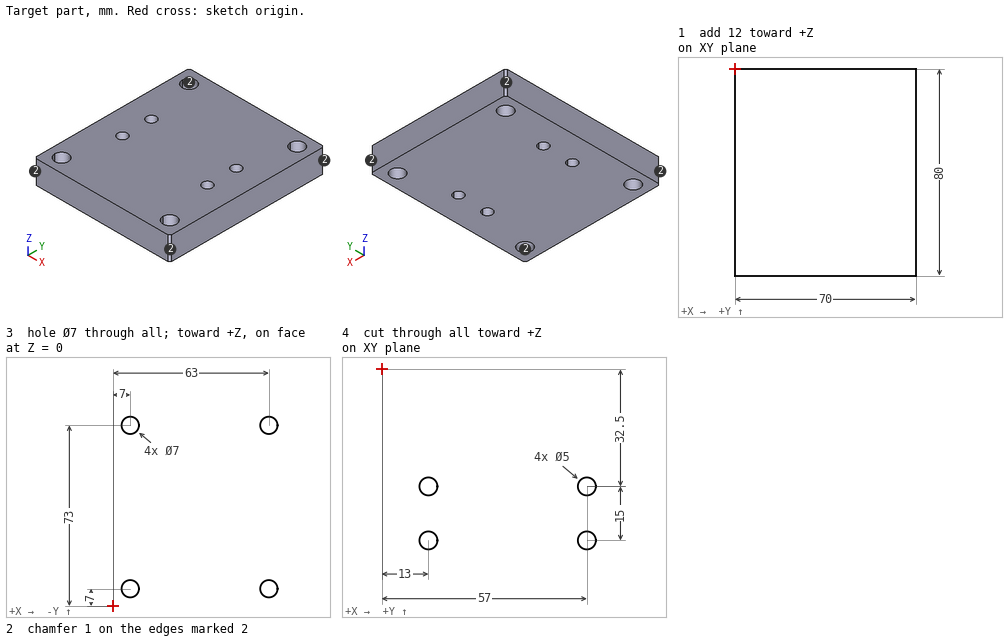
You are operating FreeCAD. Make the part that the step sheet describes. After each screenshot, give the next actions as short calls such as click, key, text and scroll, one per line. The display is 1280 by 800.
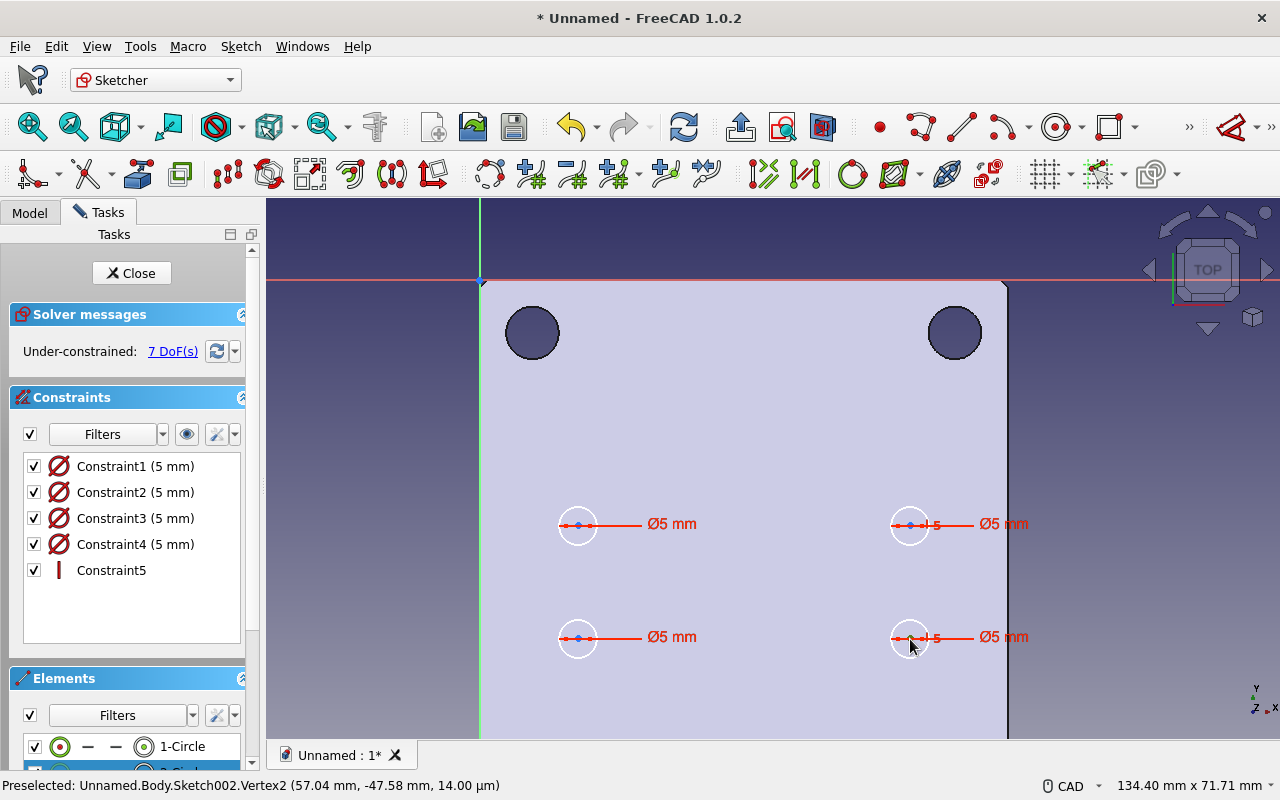
click(578, 639)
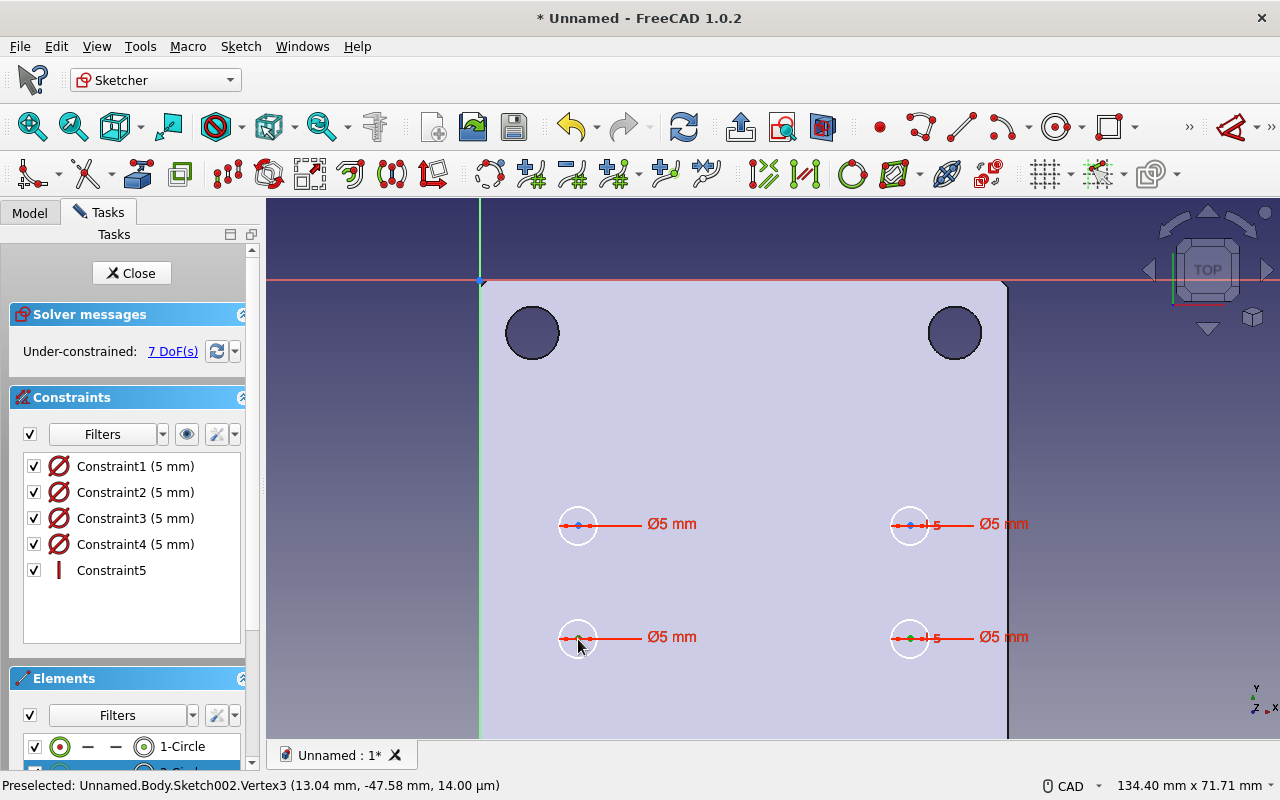
key(h)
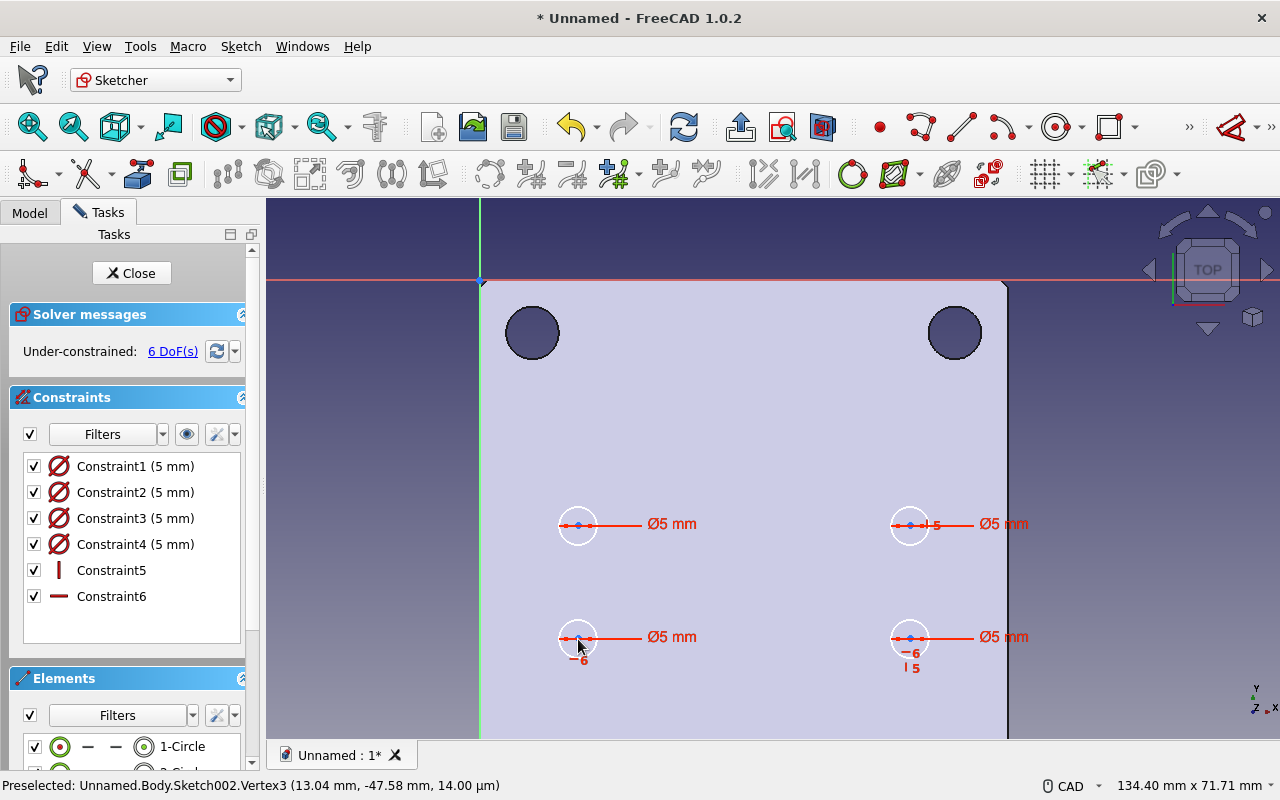
click(578, 639)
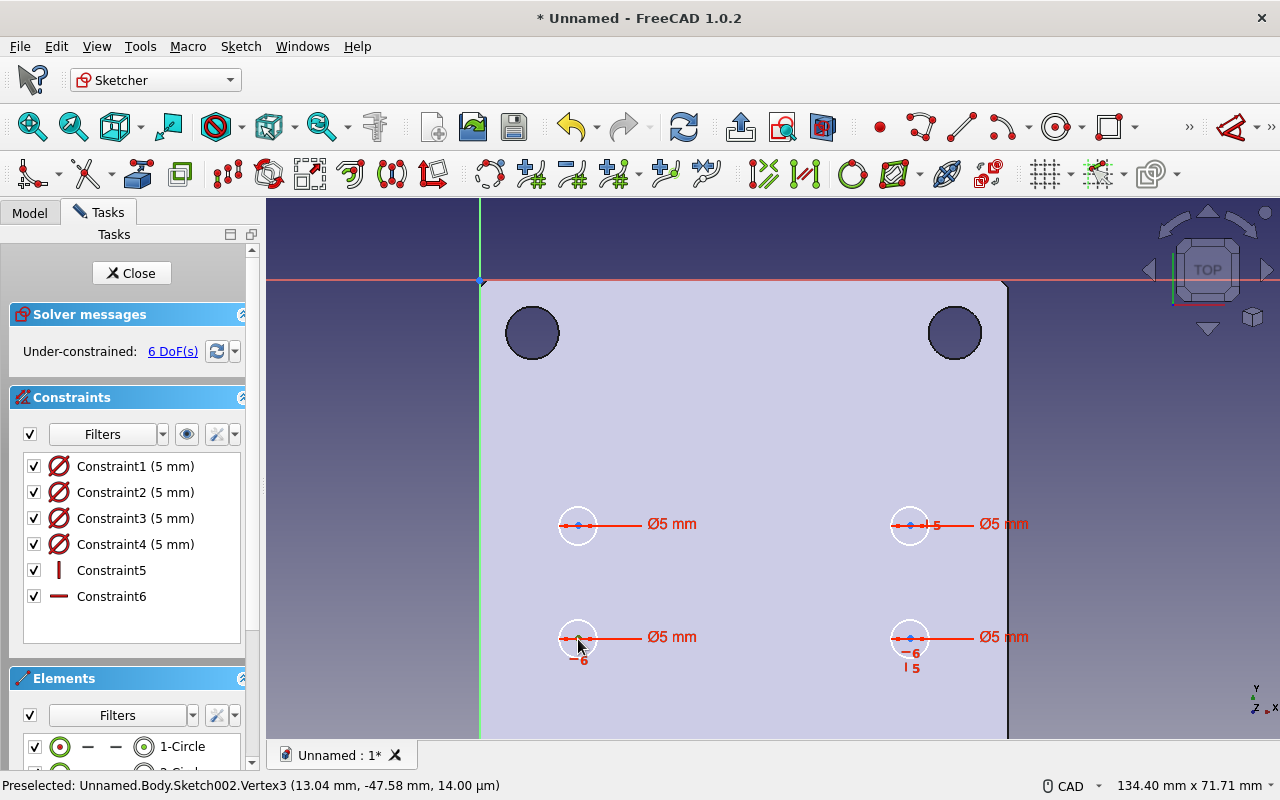
click(578, 526)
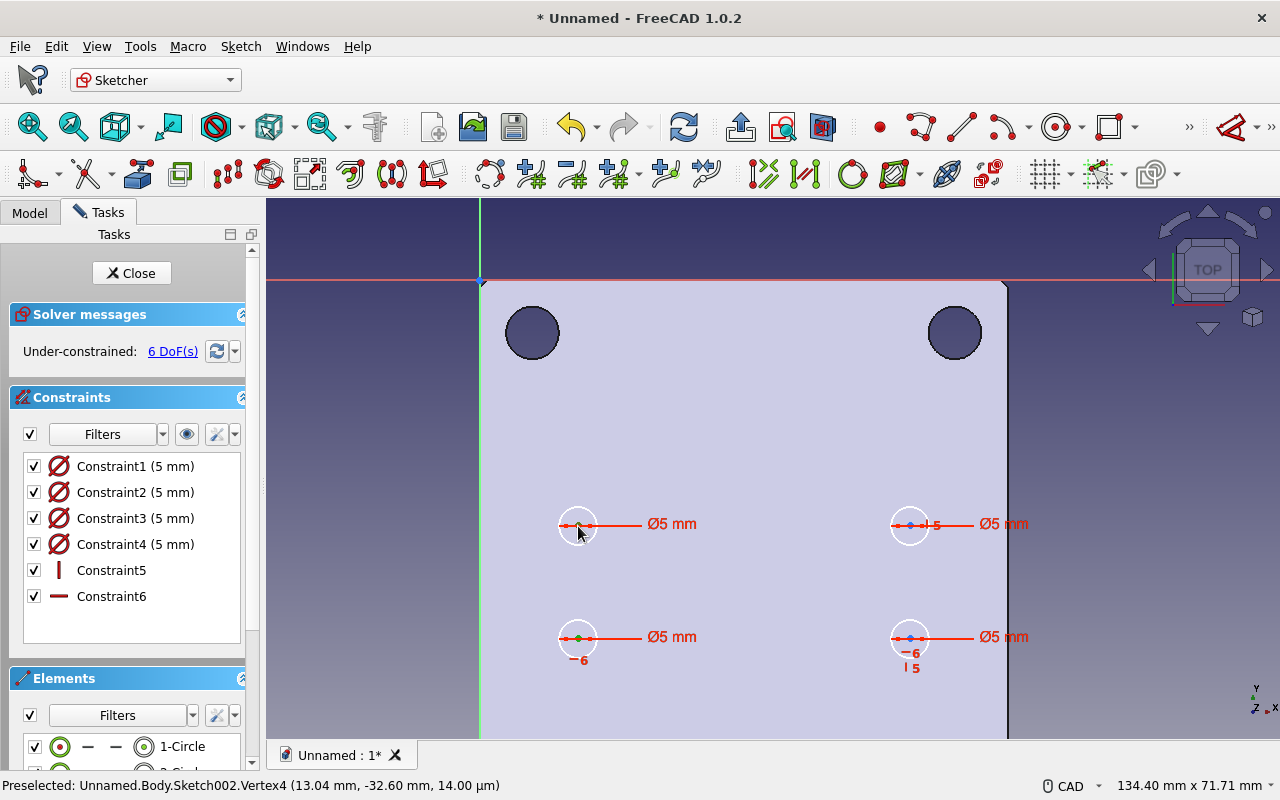
key(v)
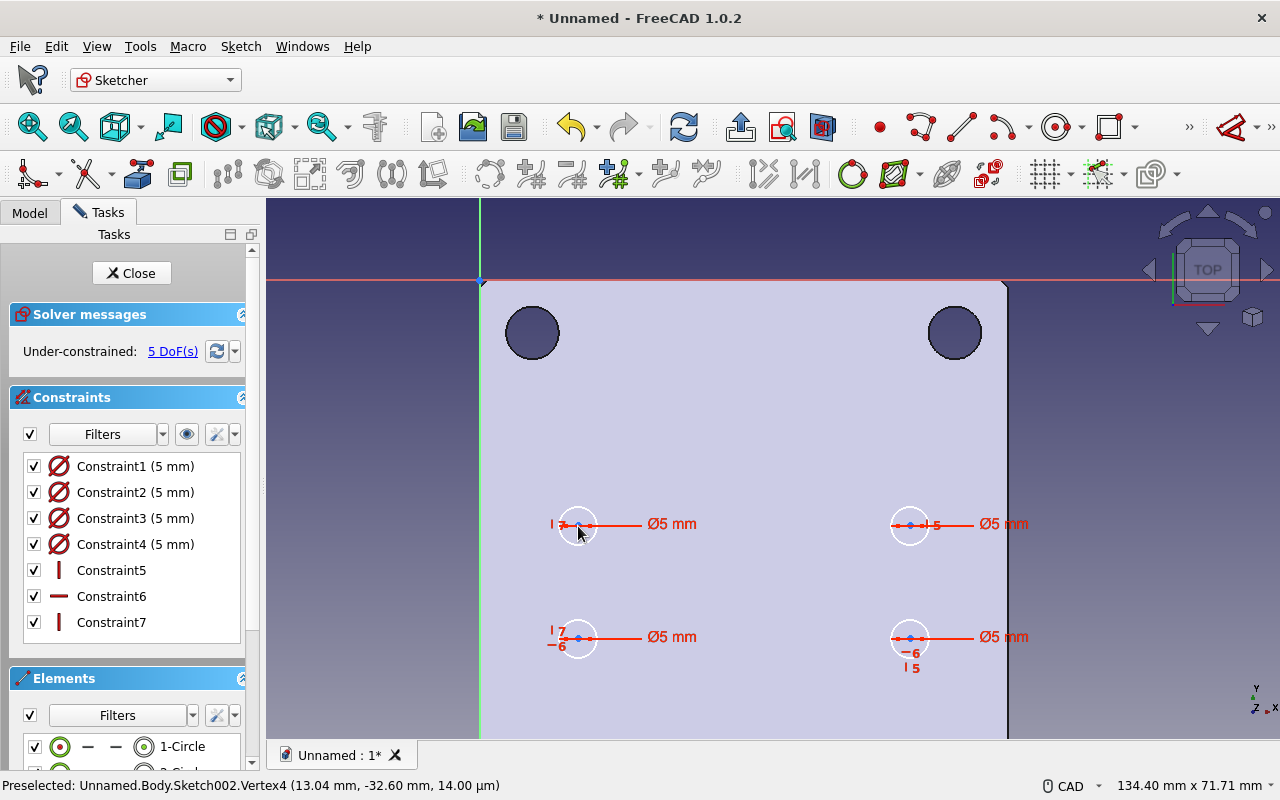
click(910, 526)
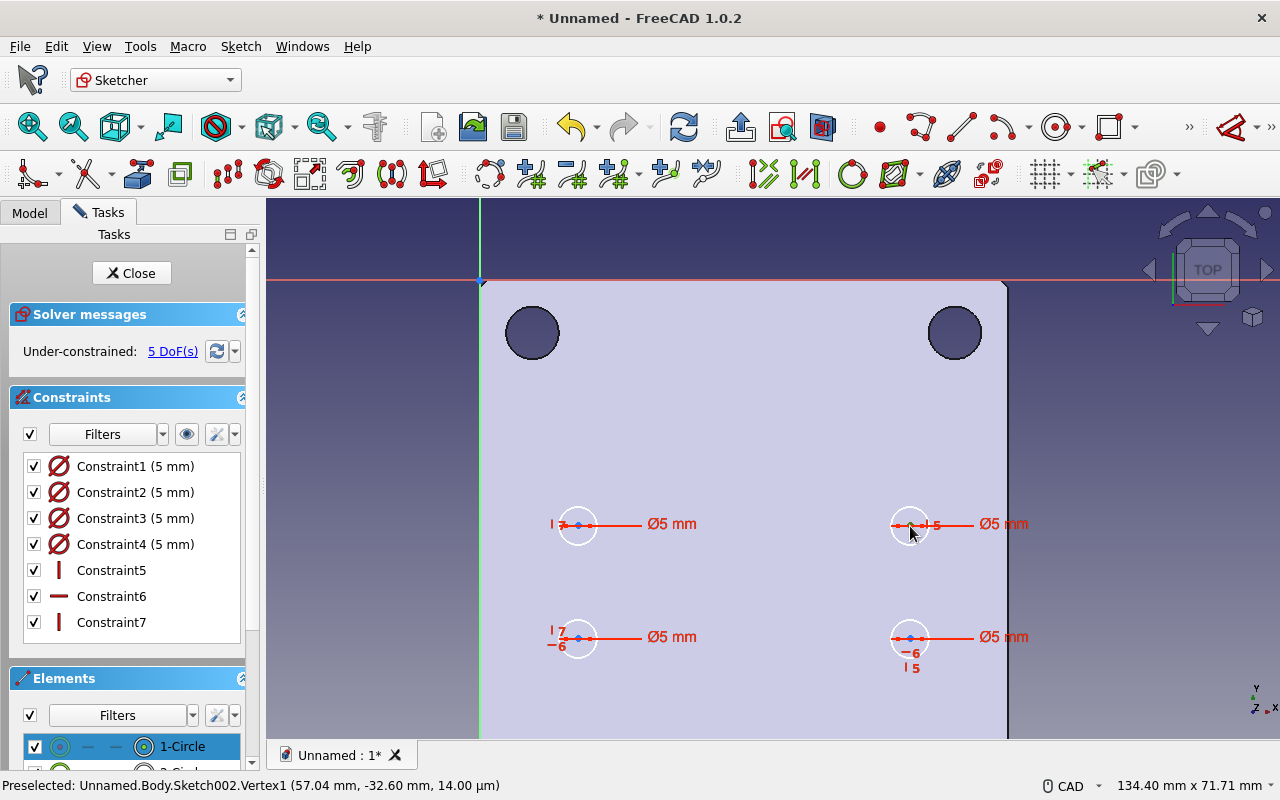
click(578, 526)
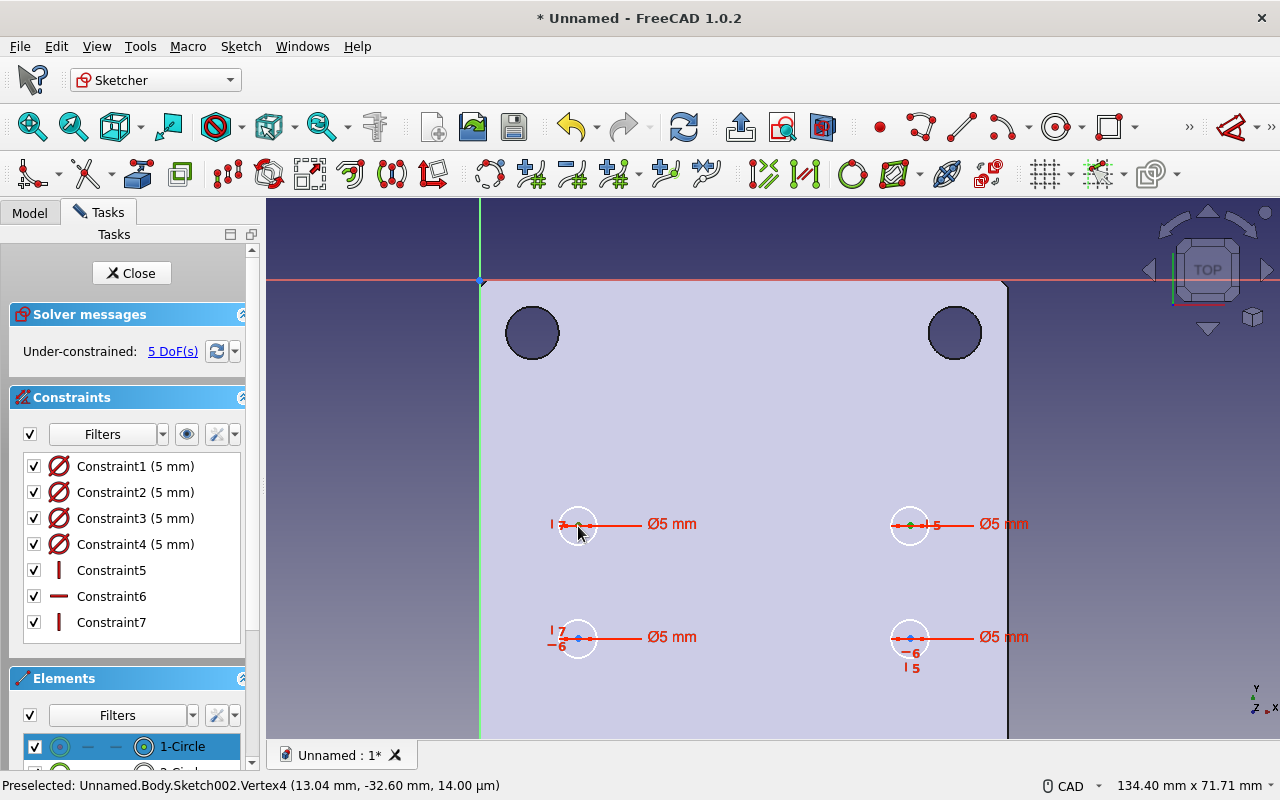
key(h)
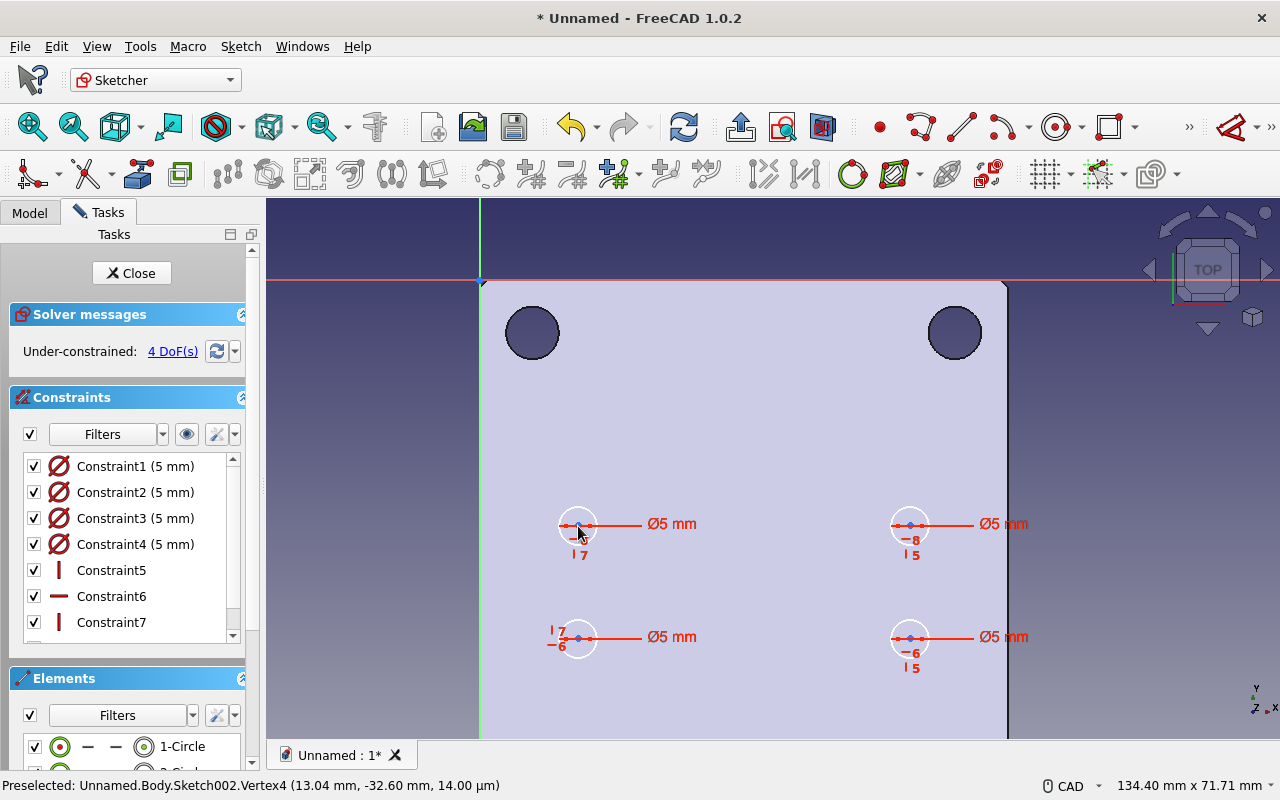
click(1230, 128)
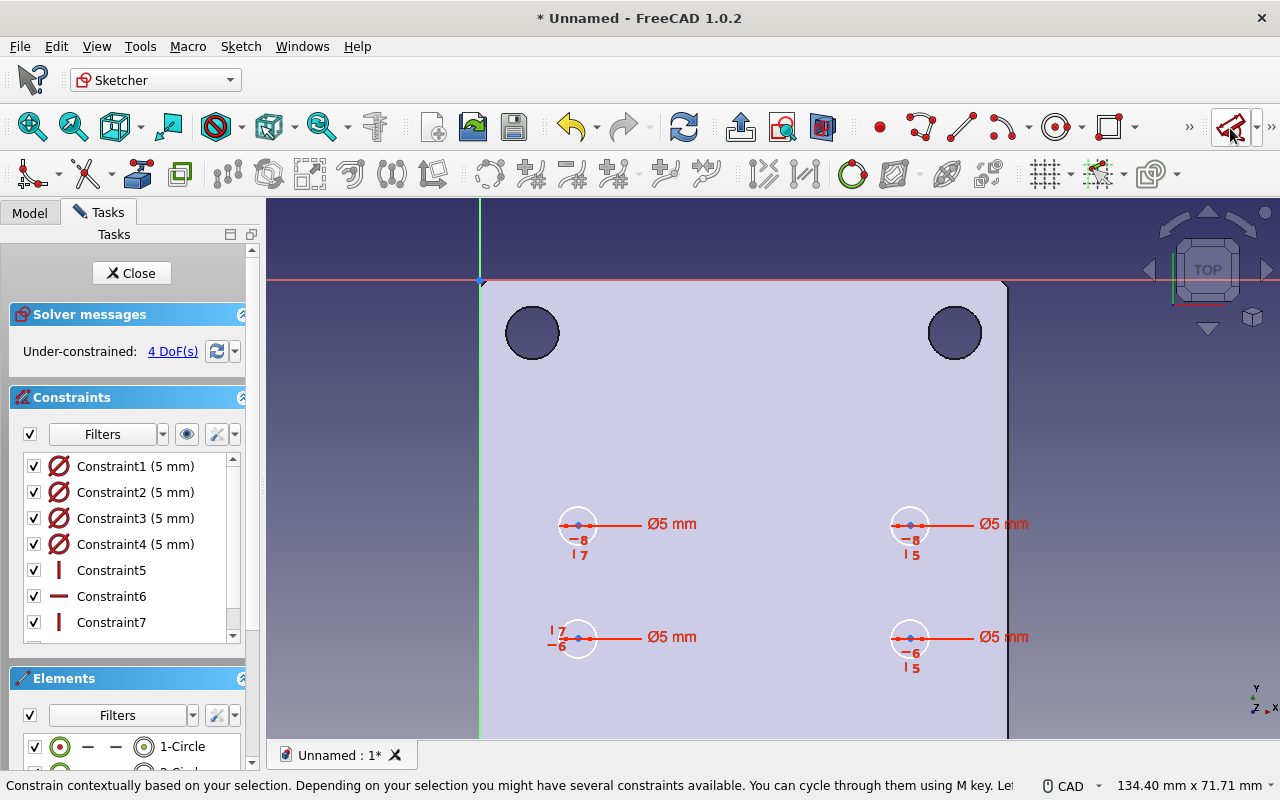
click(910, 526)
click(695, 246)